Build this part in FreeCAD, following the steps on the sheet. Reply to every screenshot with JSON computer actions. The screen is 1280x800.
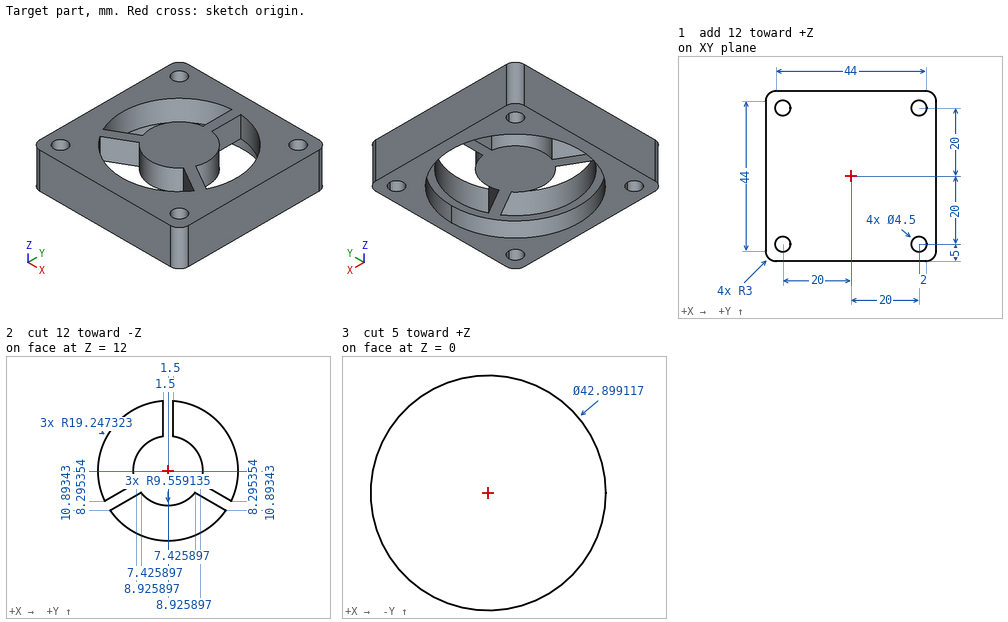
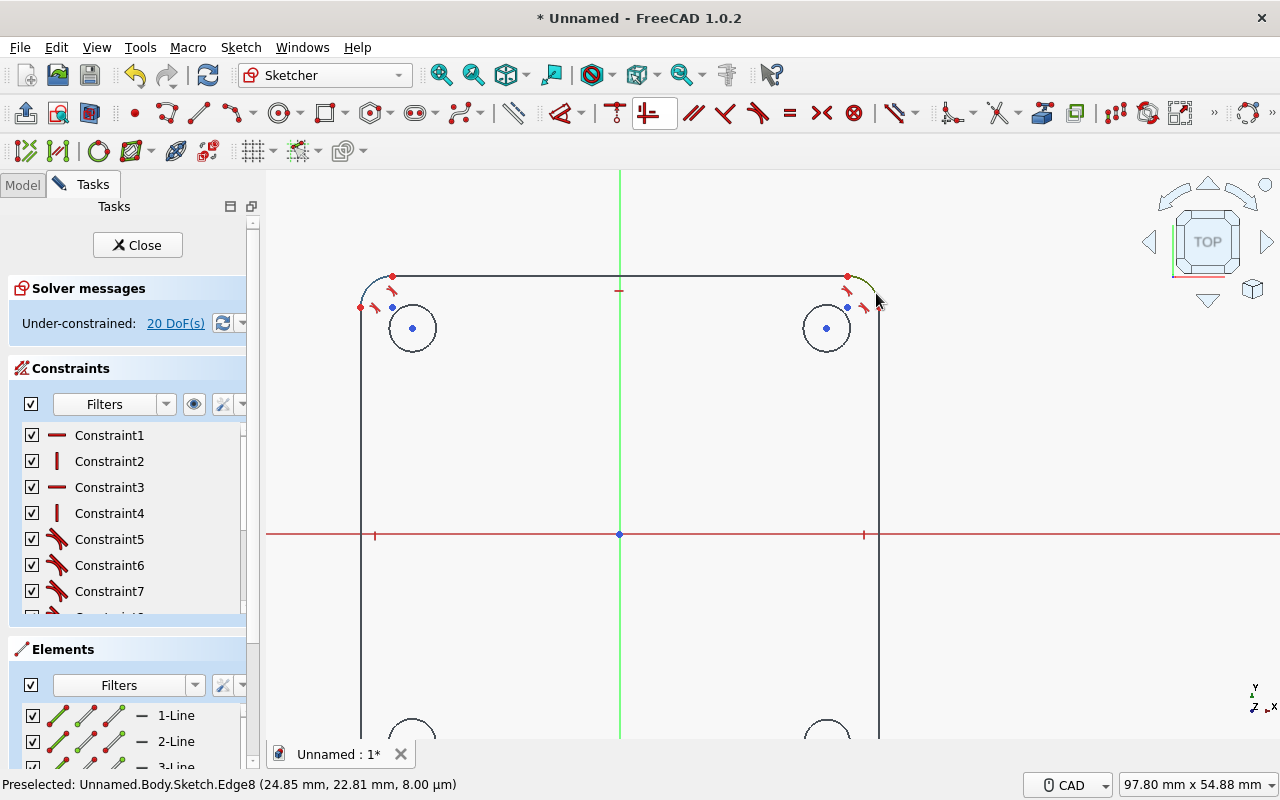
{"action": "left_click", "coordinate": [790, 114]}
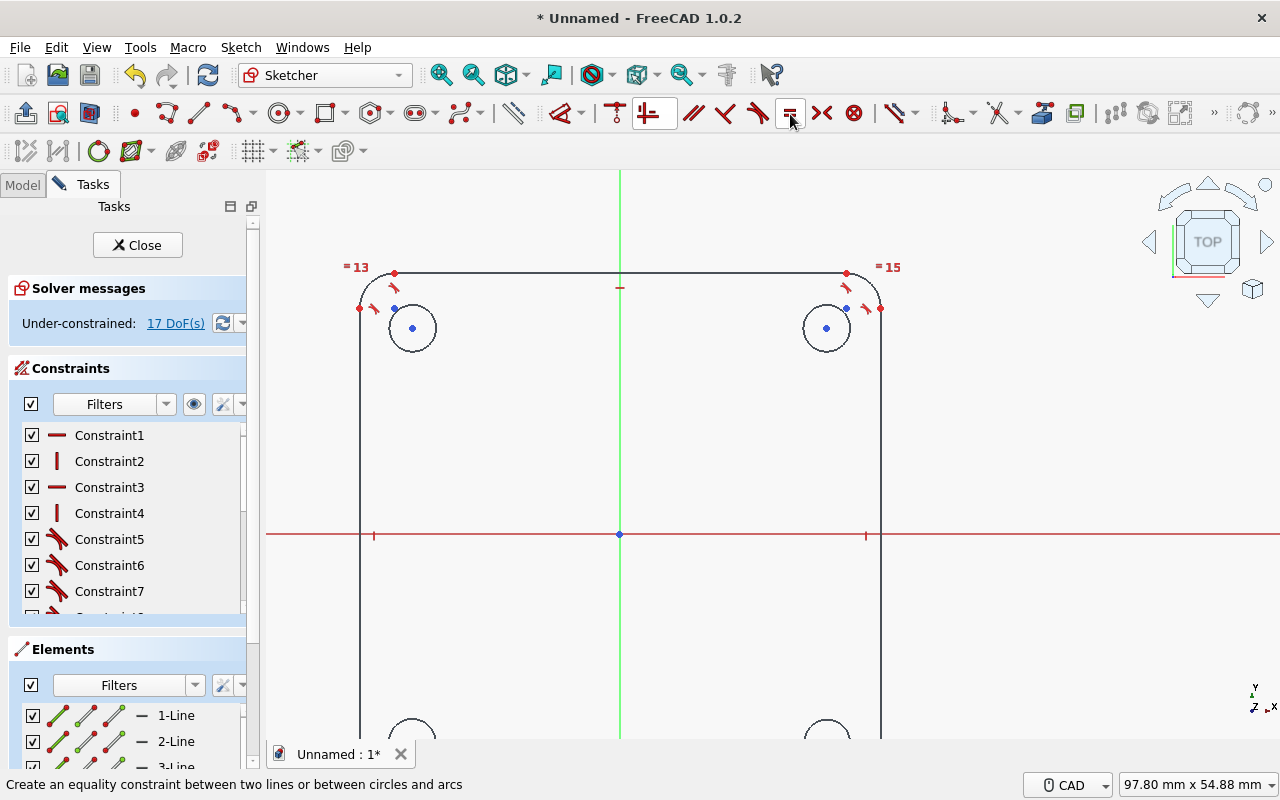
{"action": "scroll", "coordinate": [877, 292], "scroll_direction": "down", "scroll_amount": 2}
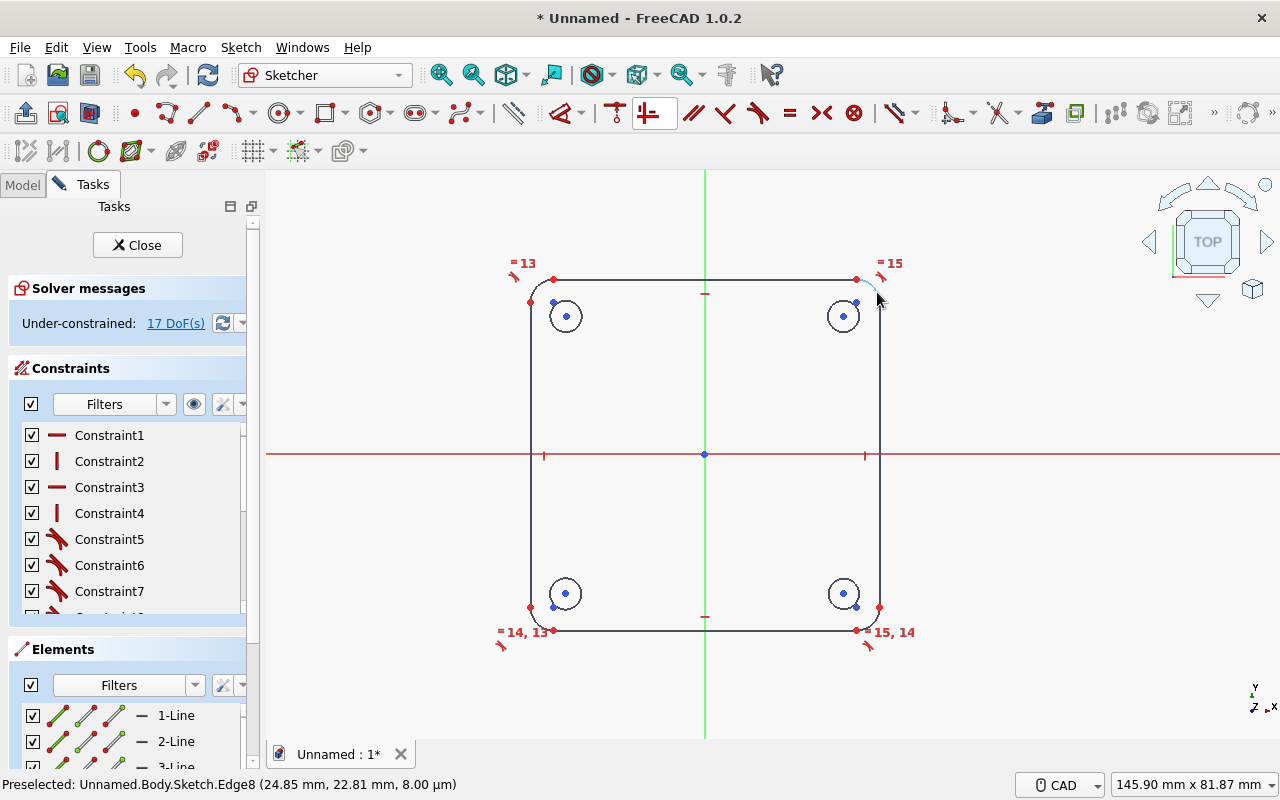
{"action": "left_click", "coordinate": [855, 583]}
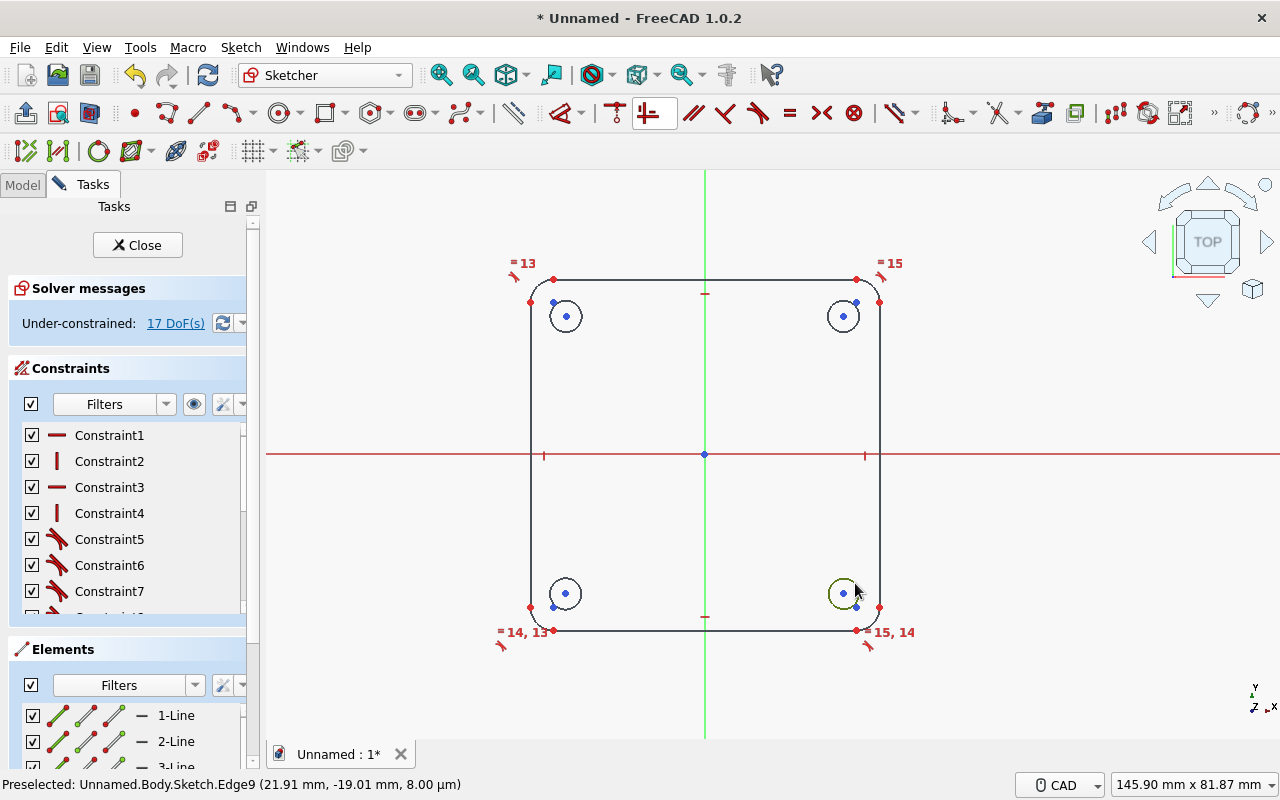
{"action": "left_click", "coordinate": [577, 583]}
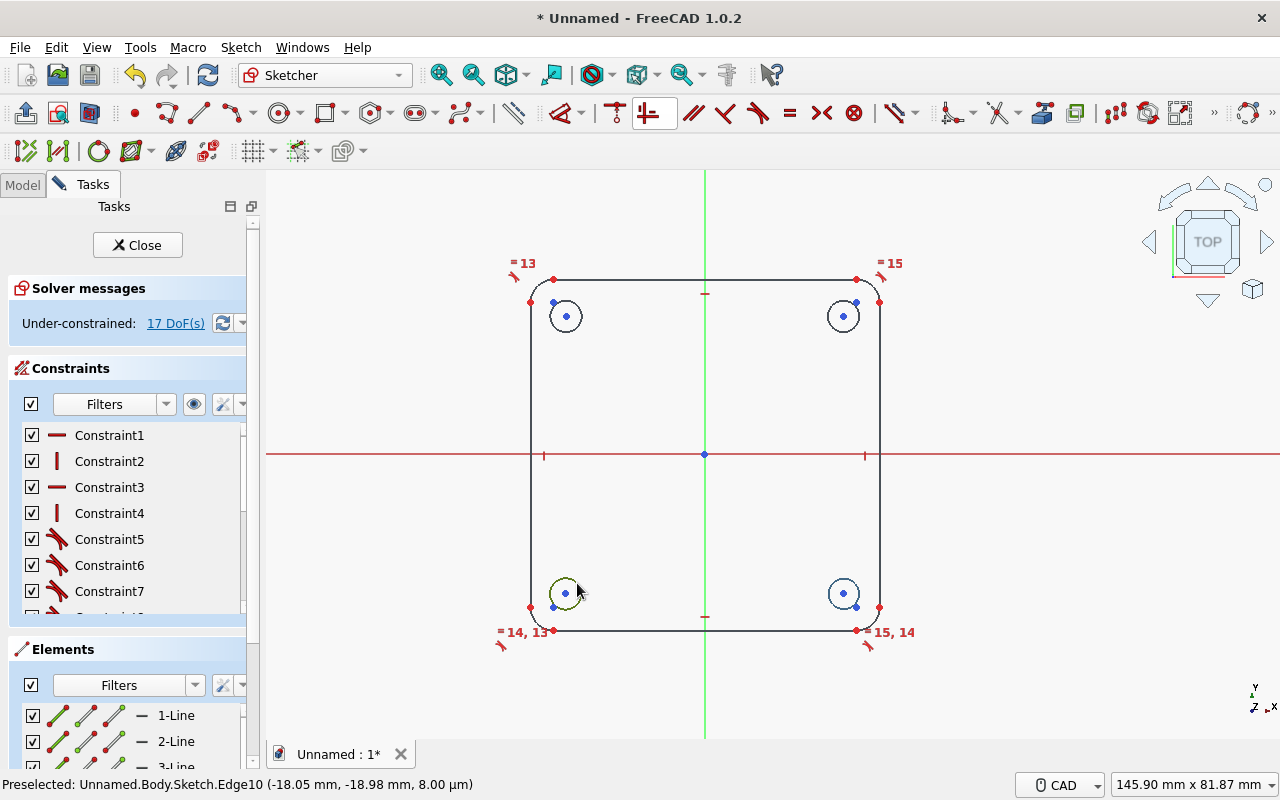
{"action": "left_click", "coordinate": [832, 305]}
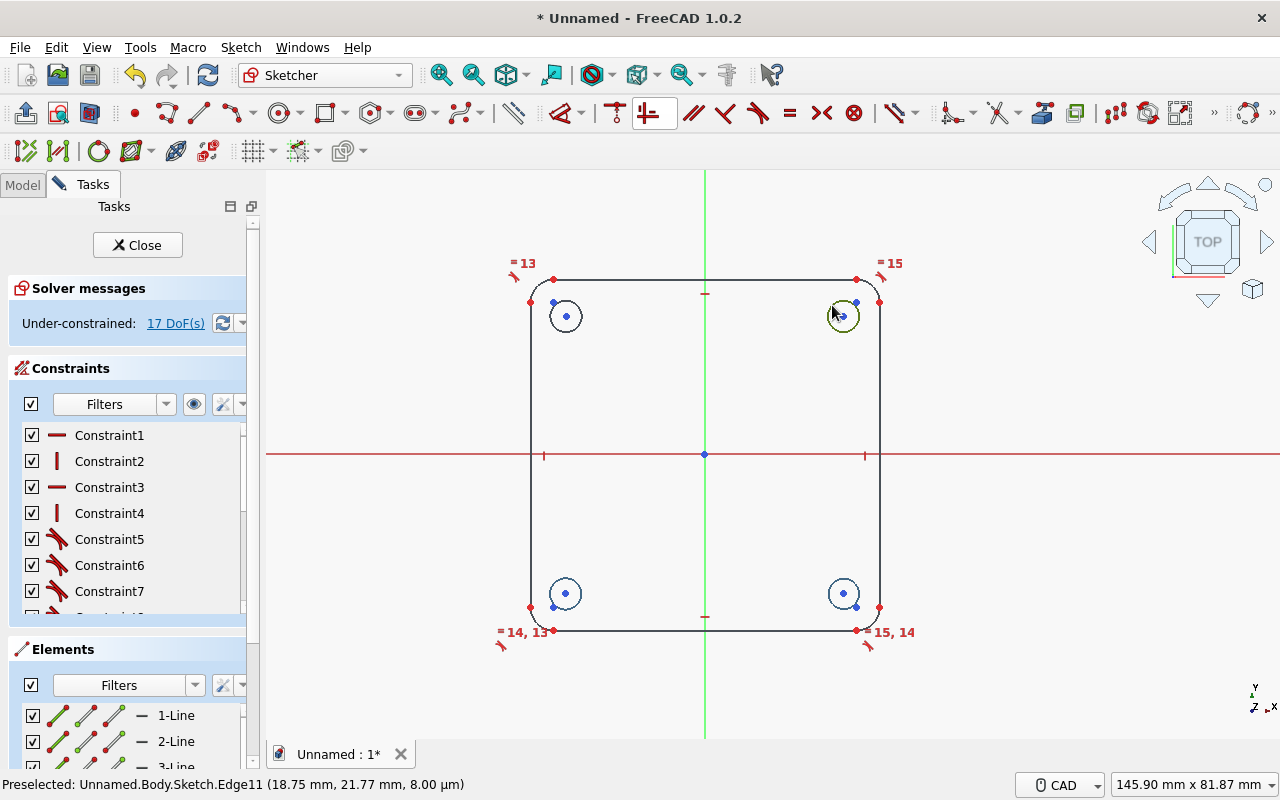
{"action": "left_click", "coordinate": [577, 305]}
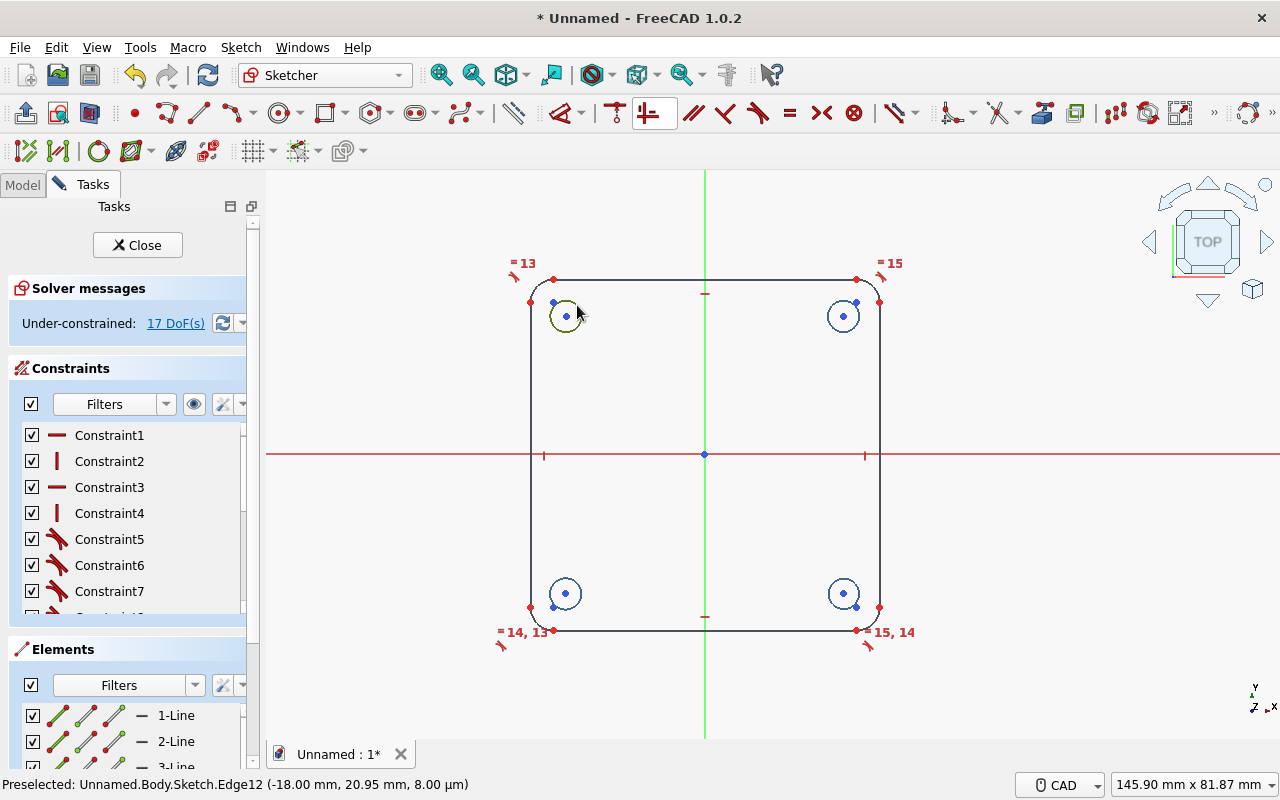
{"action": "left_click", "coordinate": [790, 114]}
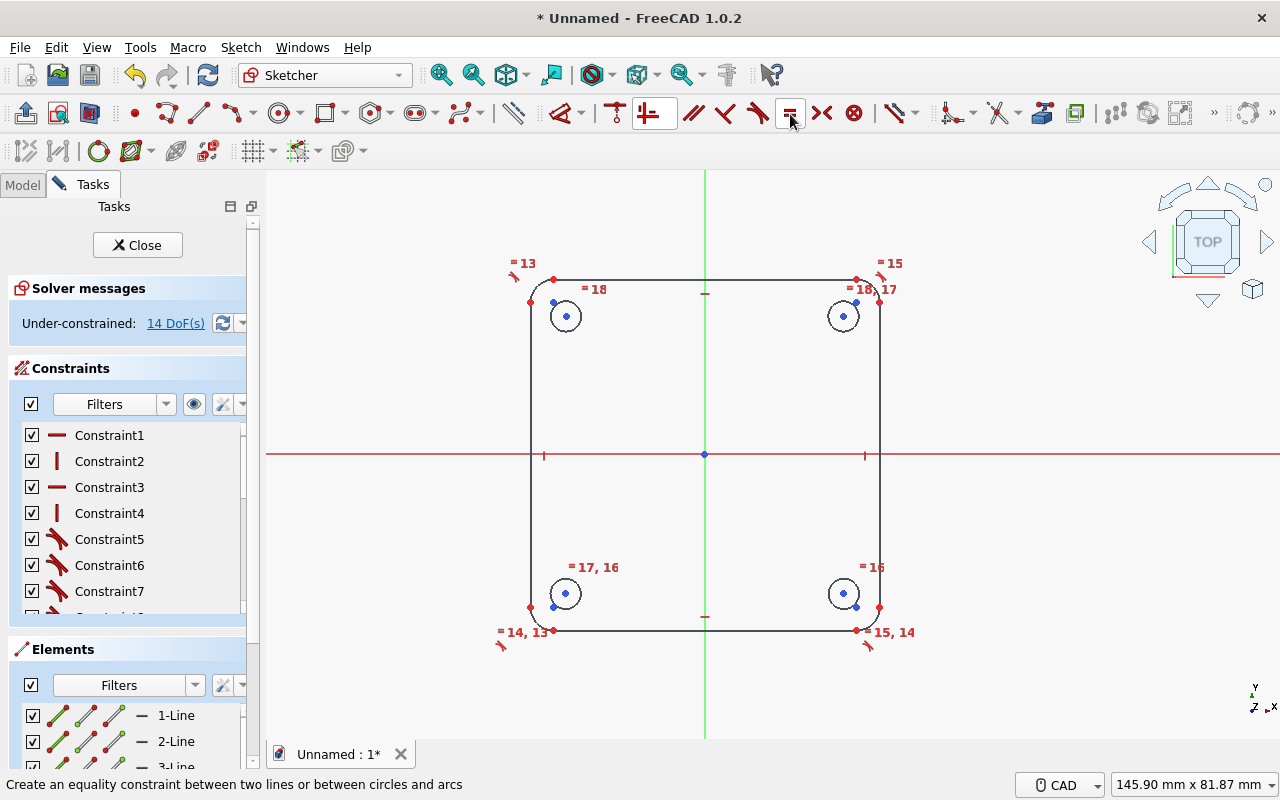
{"action": "left_click", "coordinate": [844, 594]}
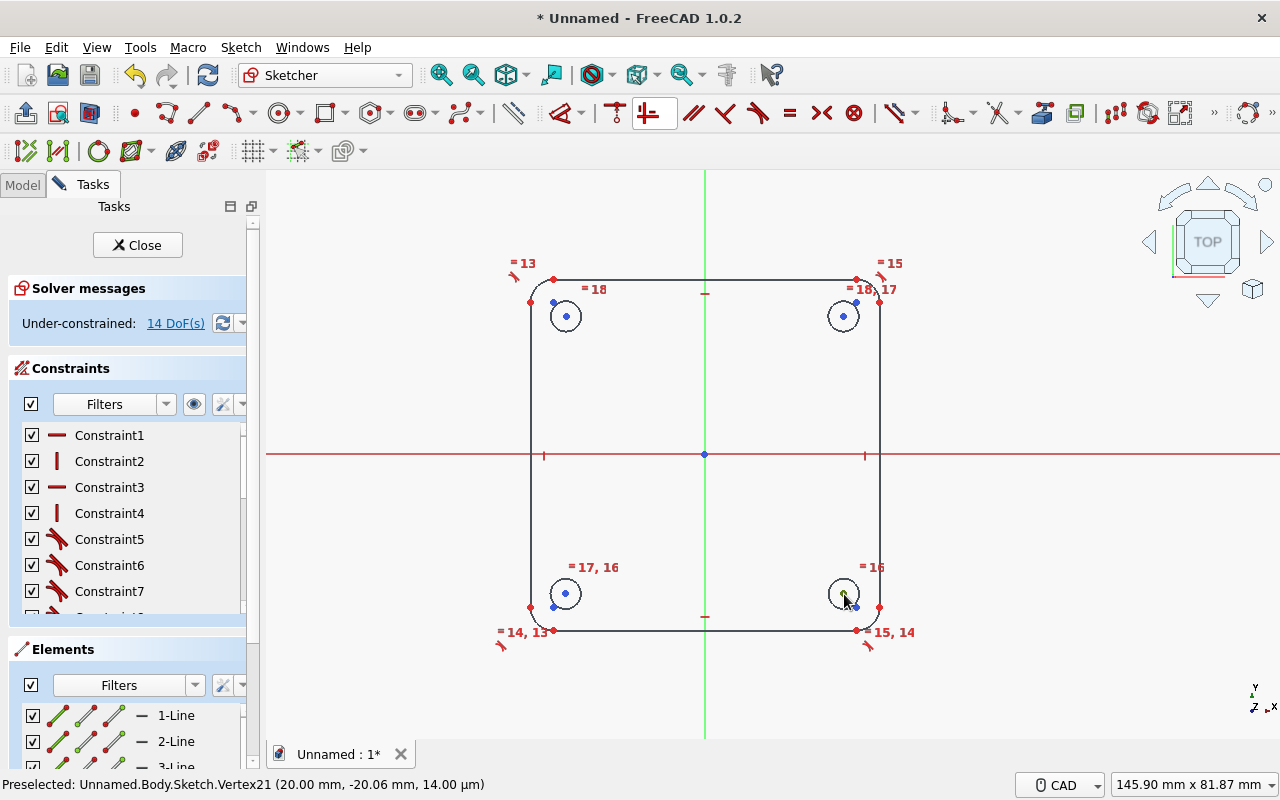
{"action": "left_click", "coordinate": [566, 594]}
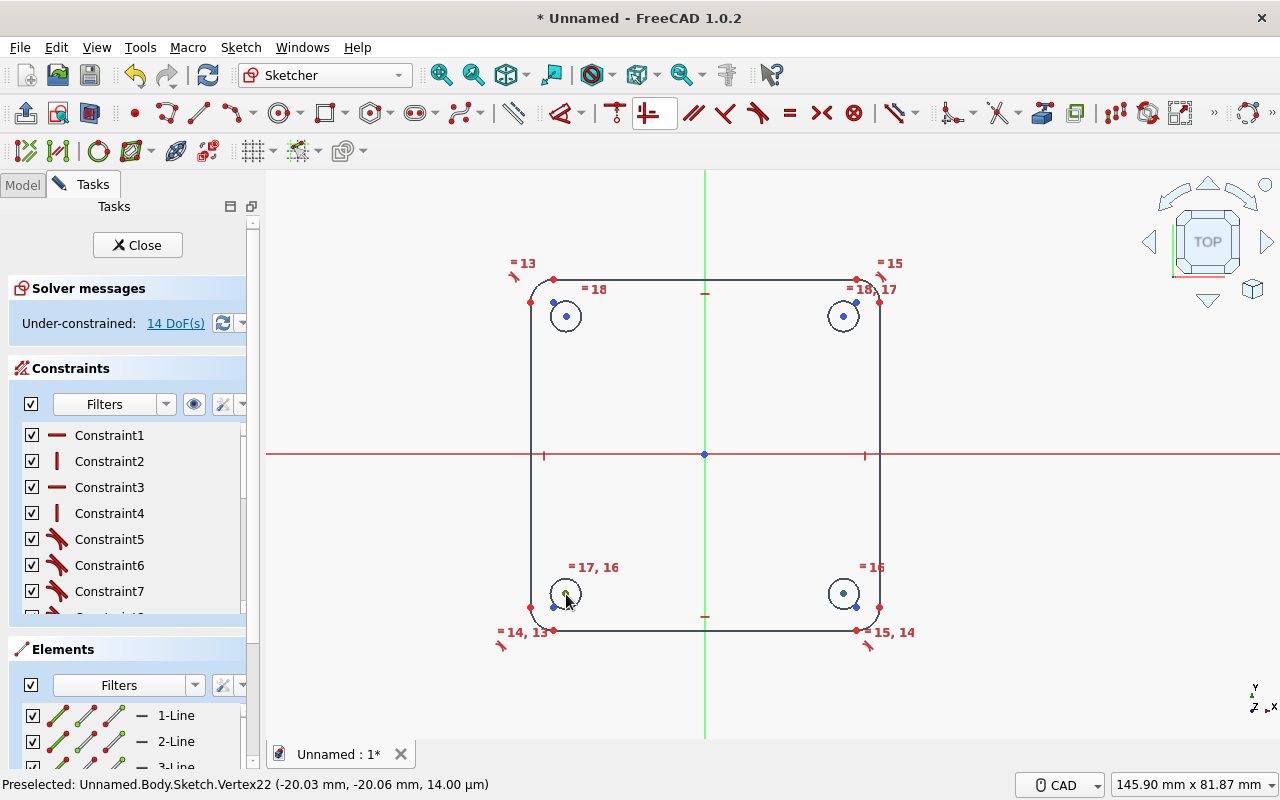
{"action": "left_click", "coordinate": [672, 114]}